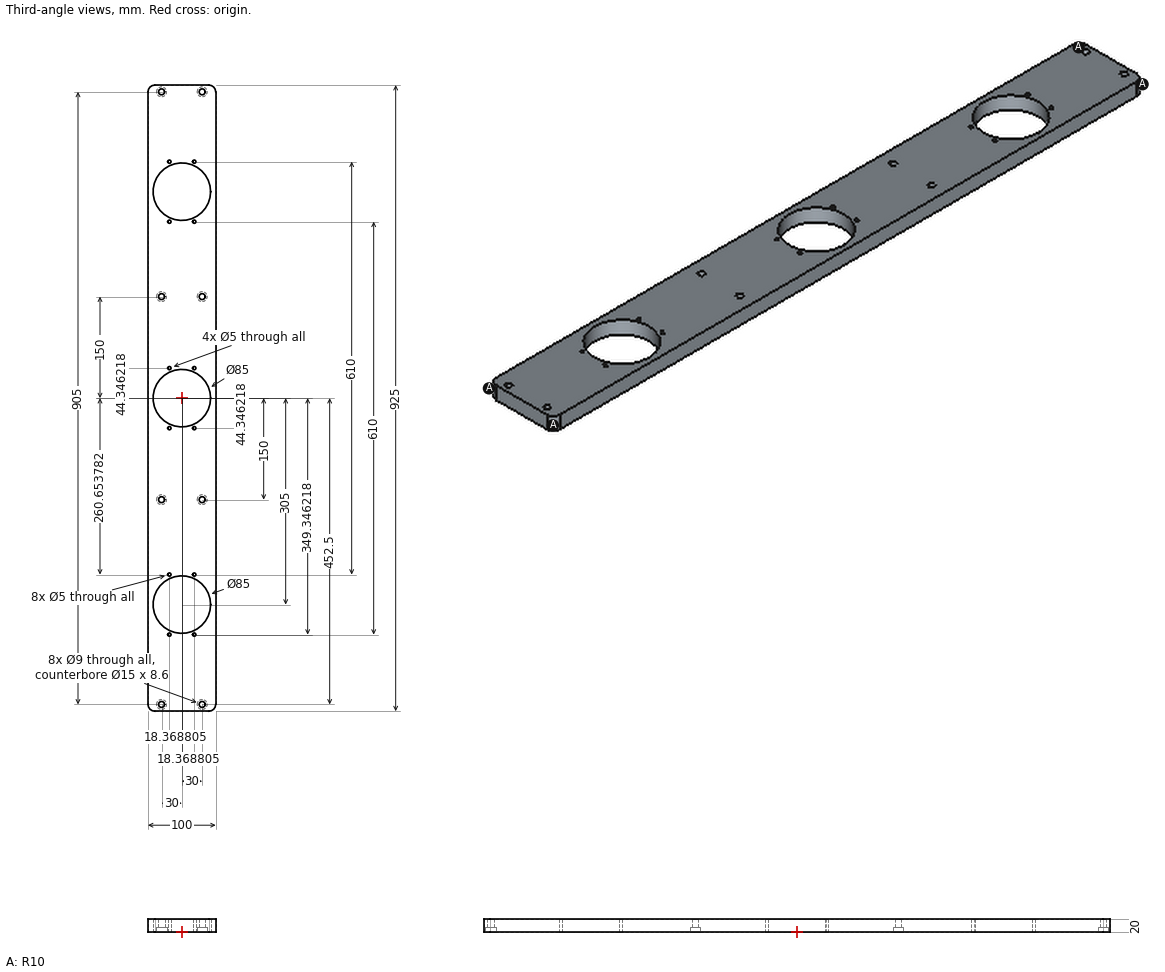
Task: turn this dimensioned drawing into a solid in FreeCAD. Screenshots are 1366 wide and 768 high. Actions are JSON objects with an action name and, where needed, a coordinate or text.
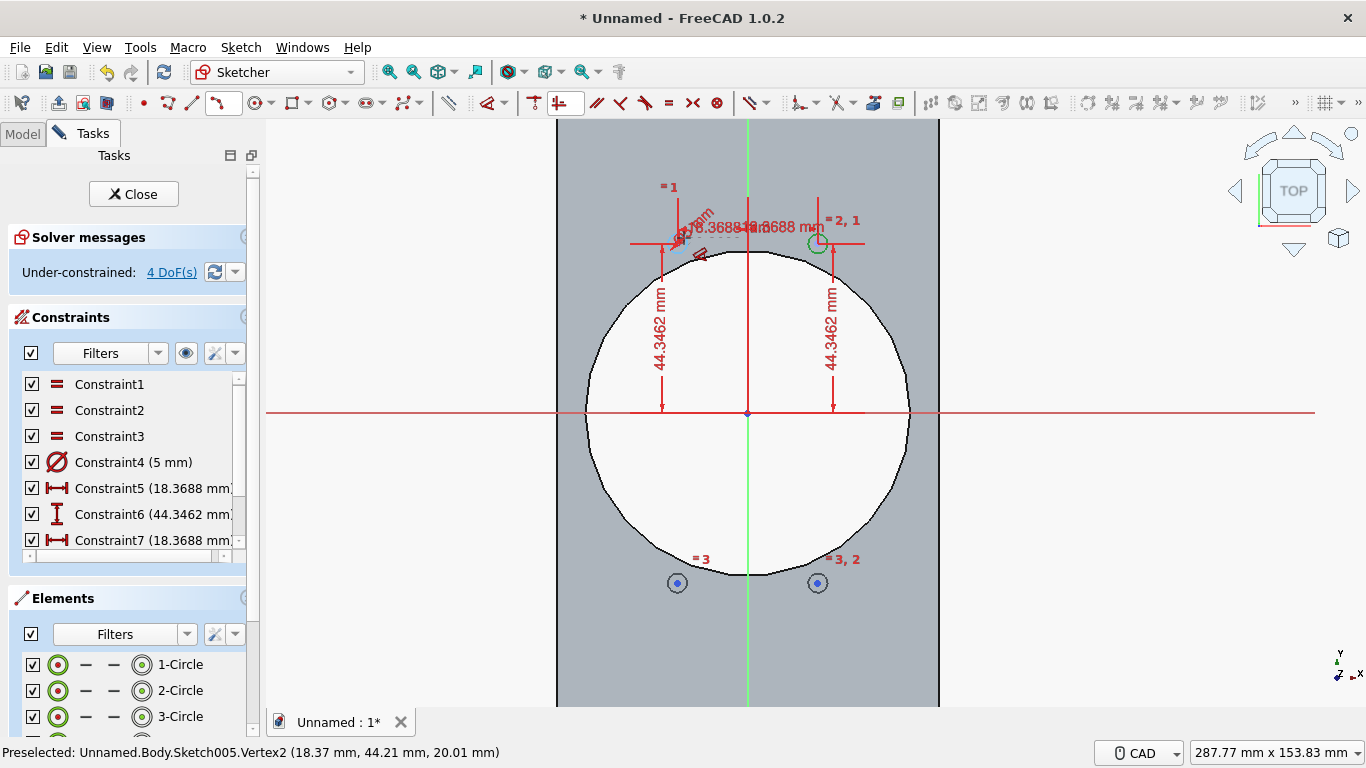
{"action": "left_click", "coordinate": [818, 583]}
{"action": "left_click", "coordinate": [783, 617]}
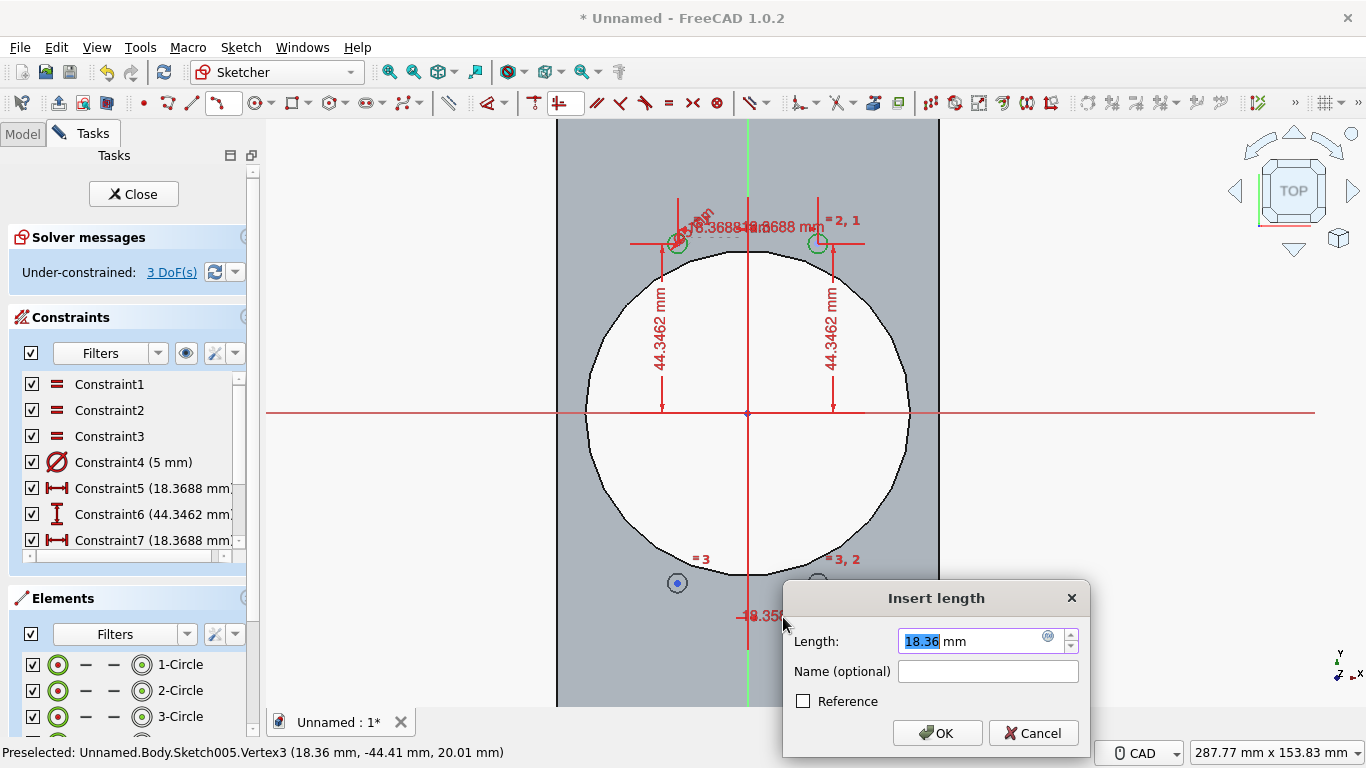
{"action": "type", "text": "18.368805"}
{"action": "key", "text": "Return"}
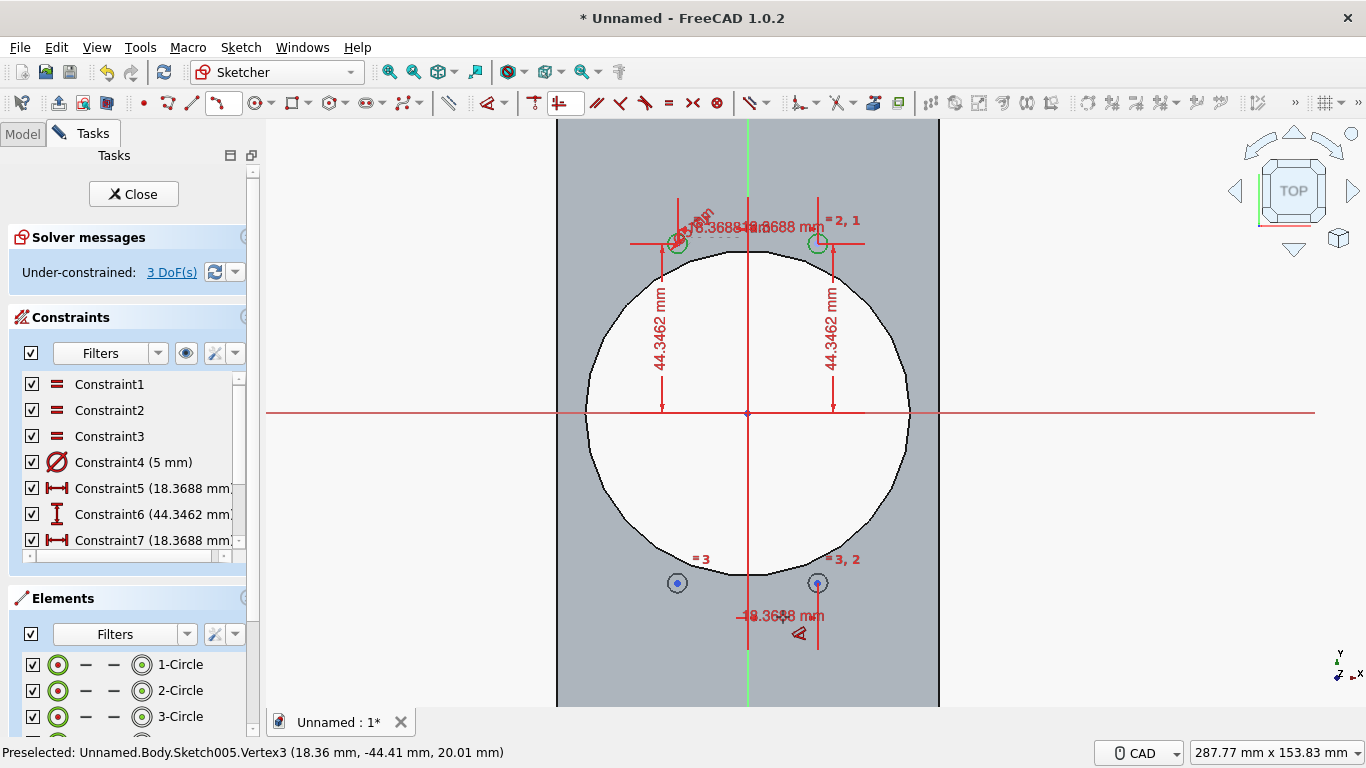
{"action": "left_click", "coordinate": [818, 583]}
{"action": "left_click", "coordinate": [852, 498]}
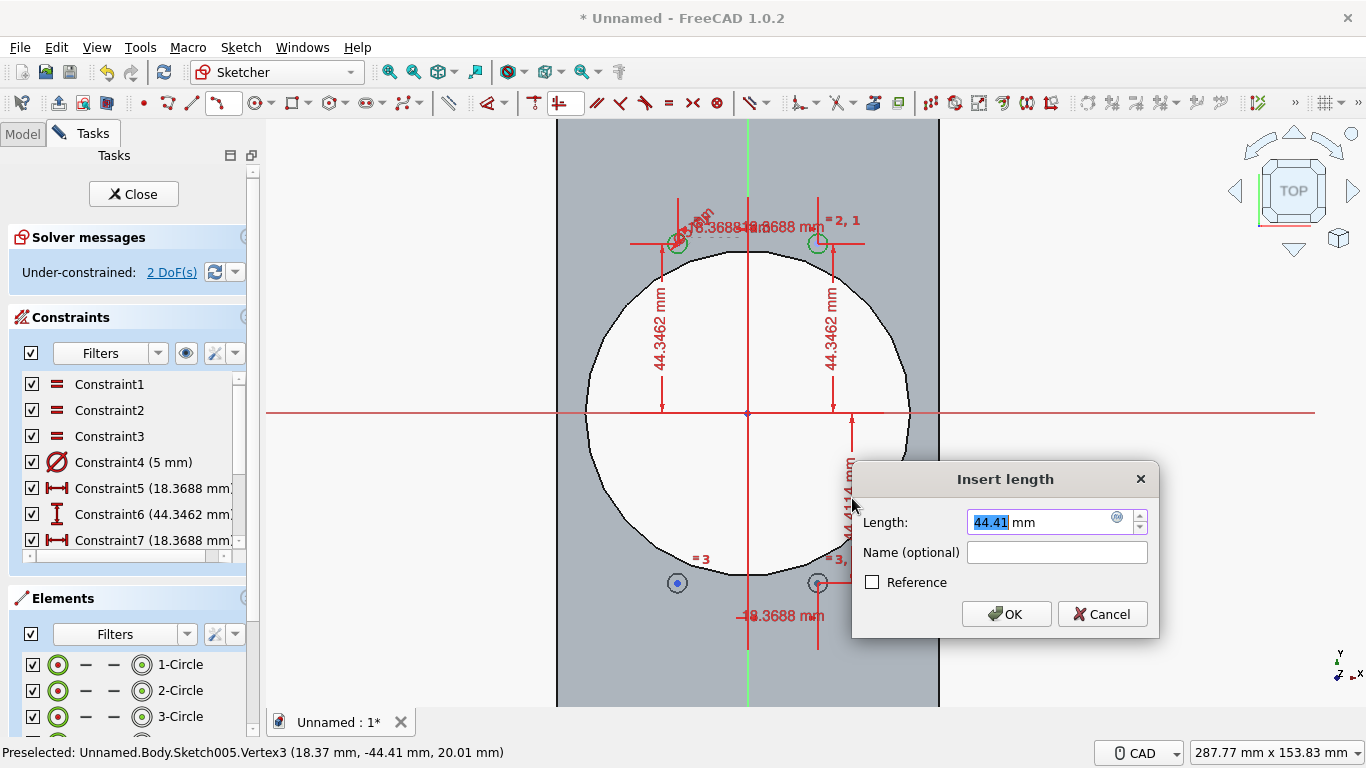
{"action": "type", "text": "44.346218"}
{"action": "key", "text": "Return"}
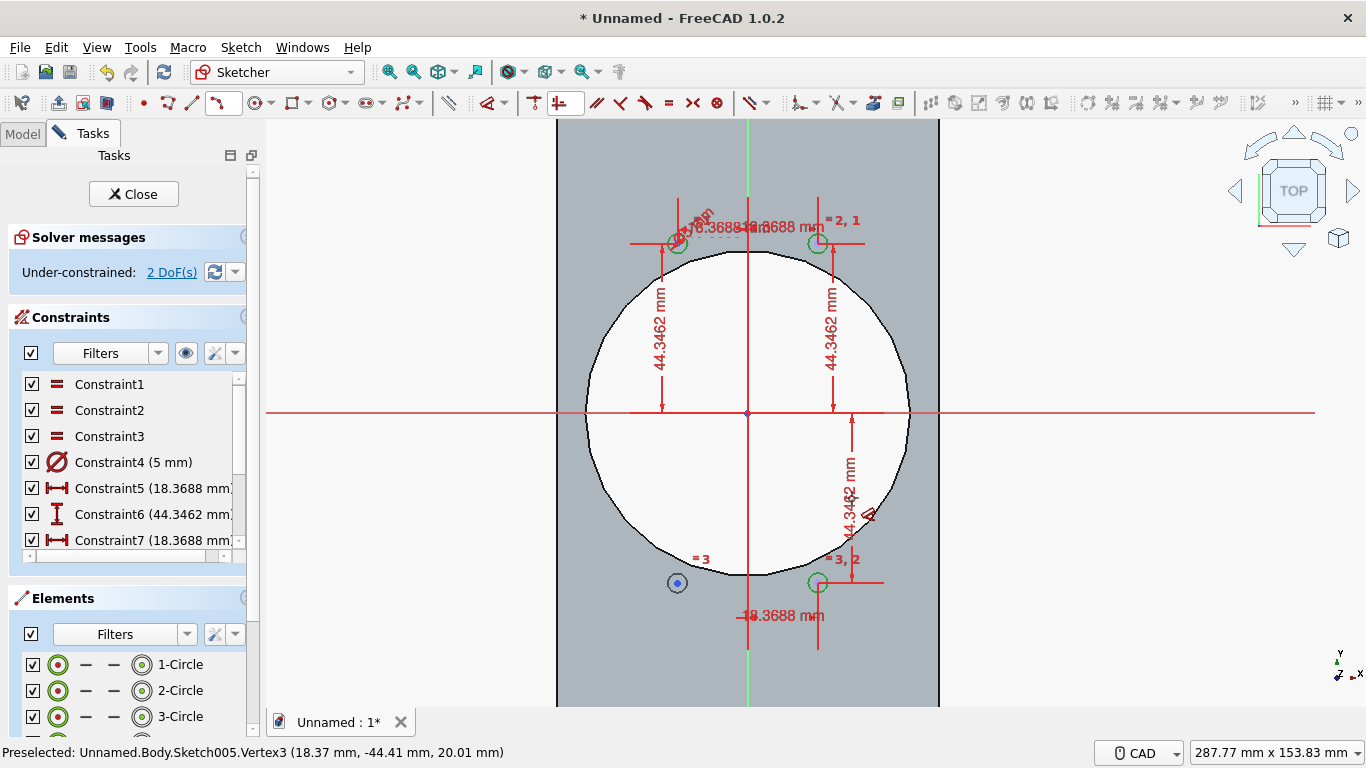
{"action": "left_click", "coordinate": [677, 583]}
{"action": "left_click", "coordinate": [713, 617]}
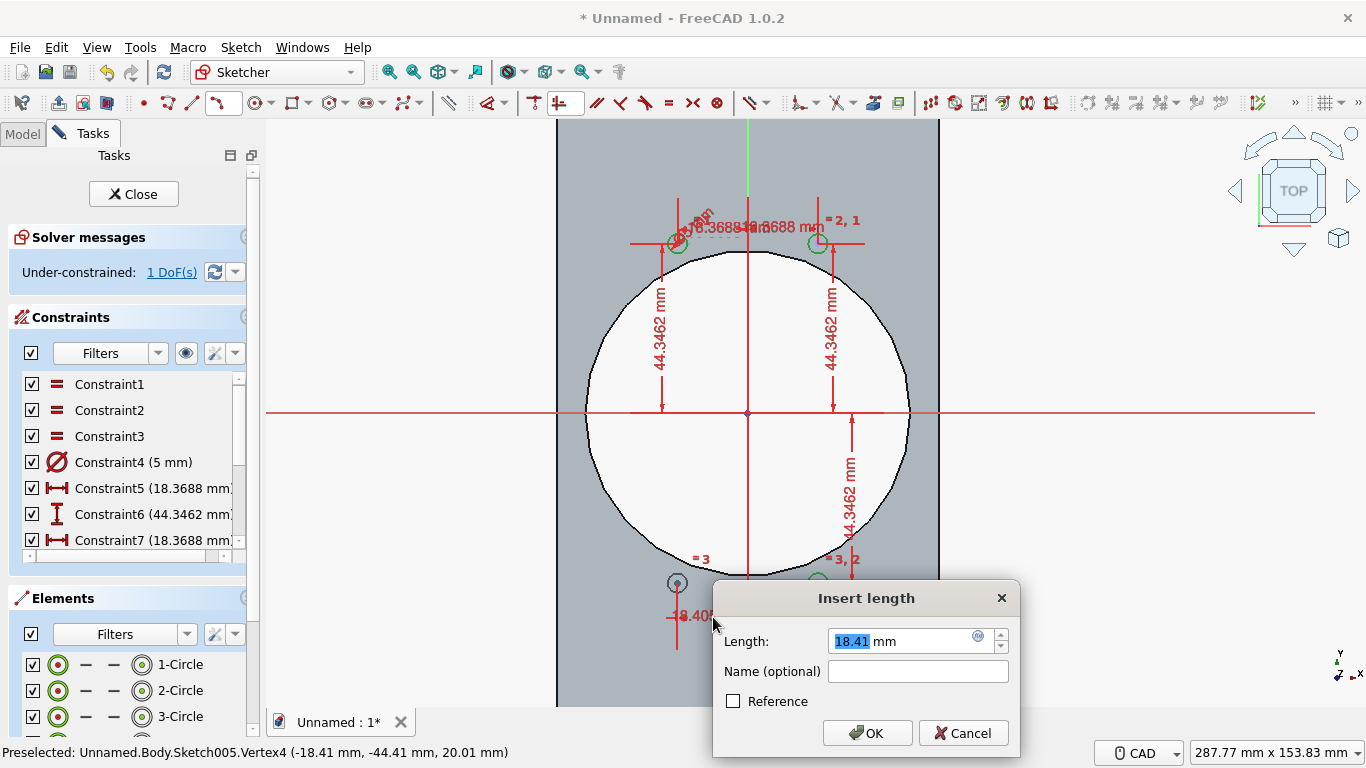
{"action": "type", "text": "18.368805"}
{"action": "key", "text": "Return"}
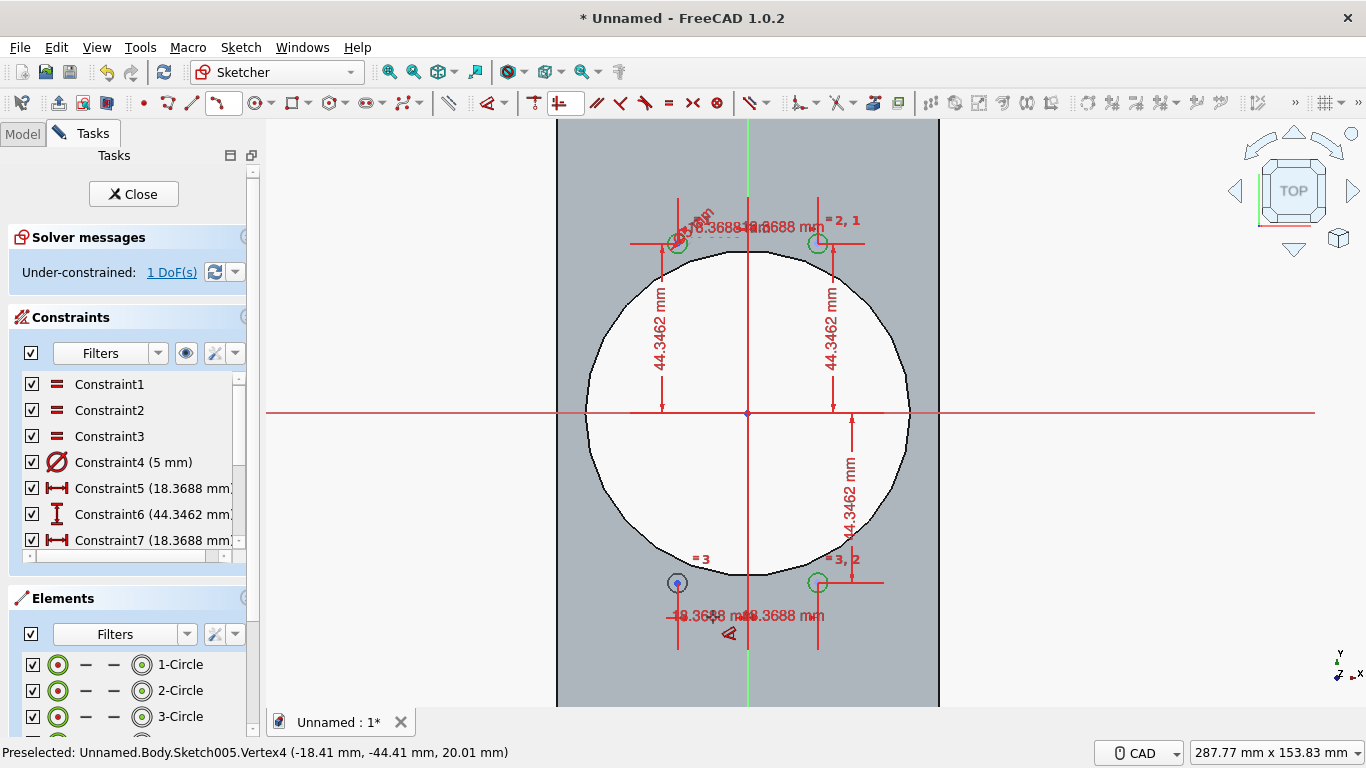
{"action": "left_click", "coordinate": [678, 583]}
{"action": "left_click", "coordinate": [644, 498]}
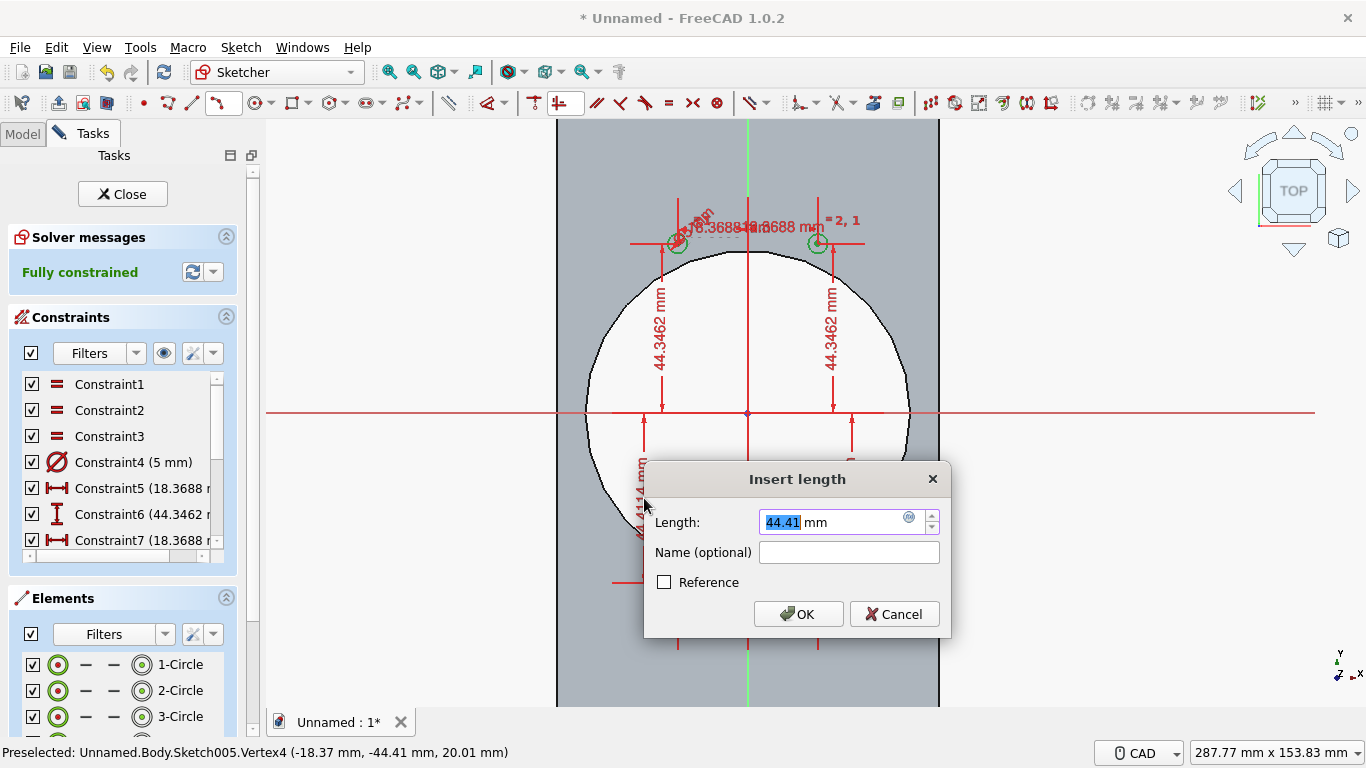
{"action": "type", "text": "44.346218"}
{"action": "key", "text": "Return"}
{"action": "key", "text": "Escape"}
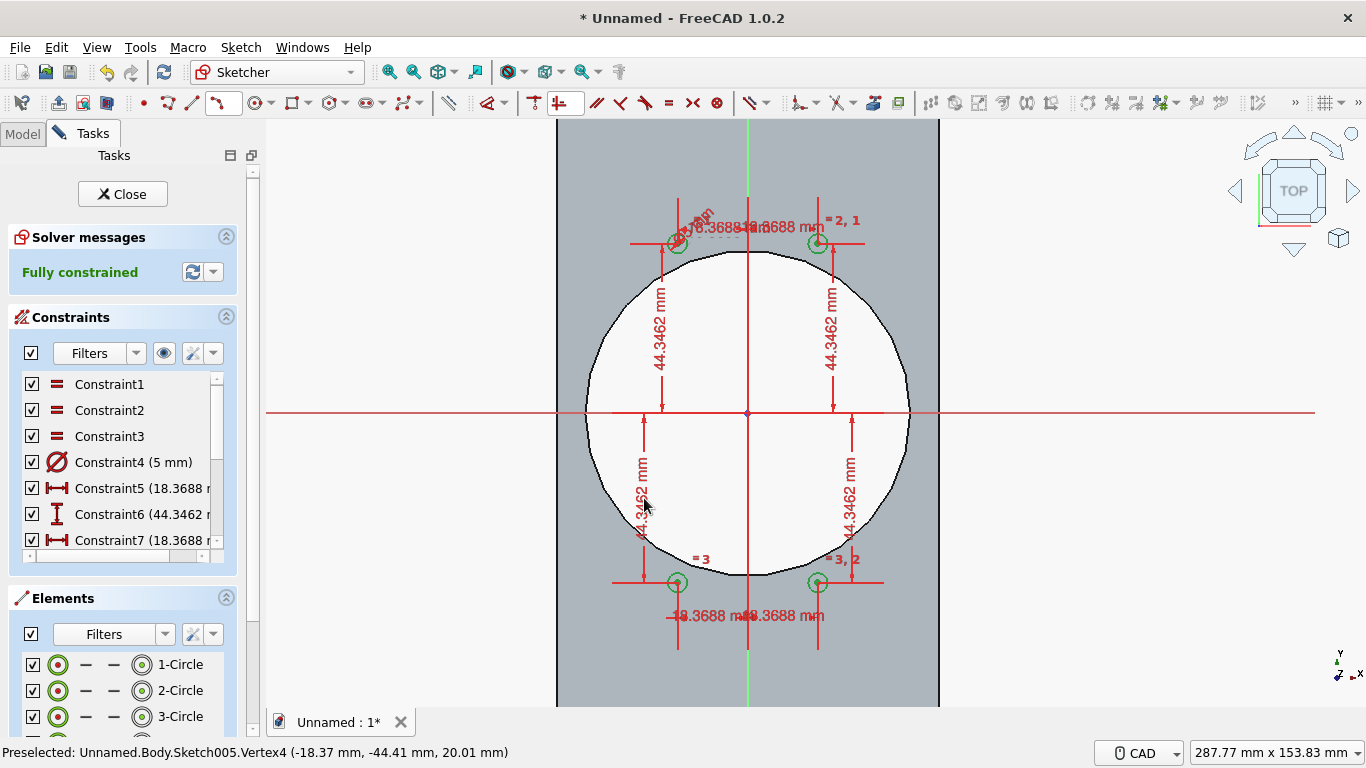
{"action": "left_click", "coordinate": [123, 194]}